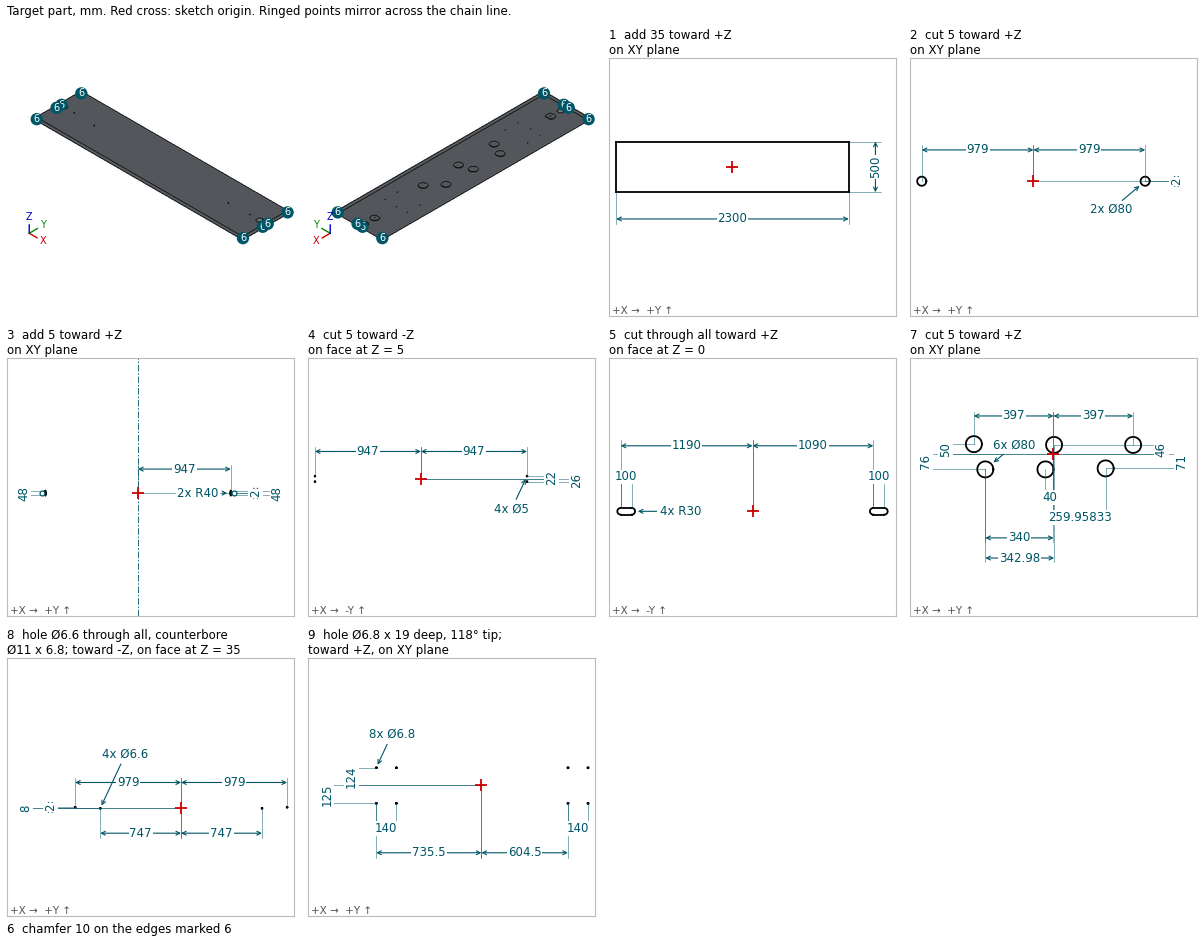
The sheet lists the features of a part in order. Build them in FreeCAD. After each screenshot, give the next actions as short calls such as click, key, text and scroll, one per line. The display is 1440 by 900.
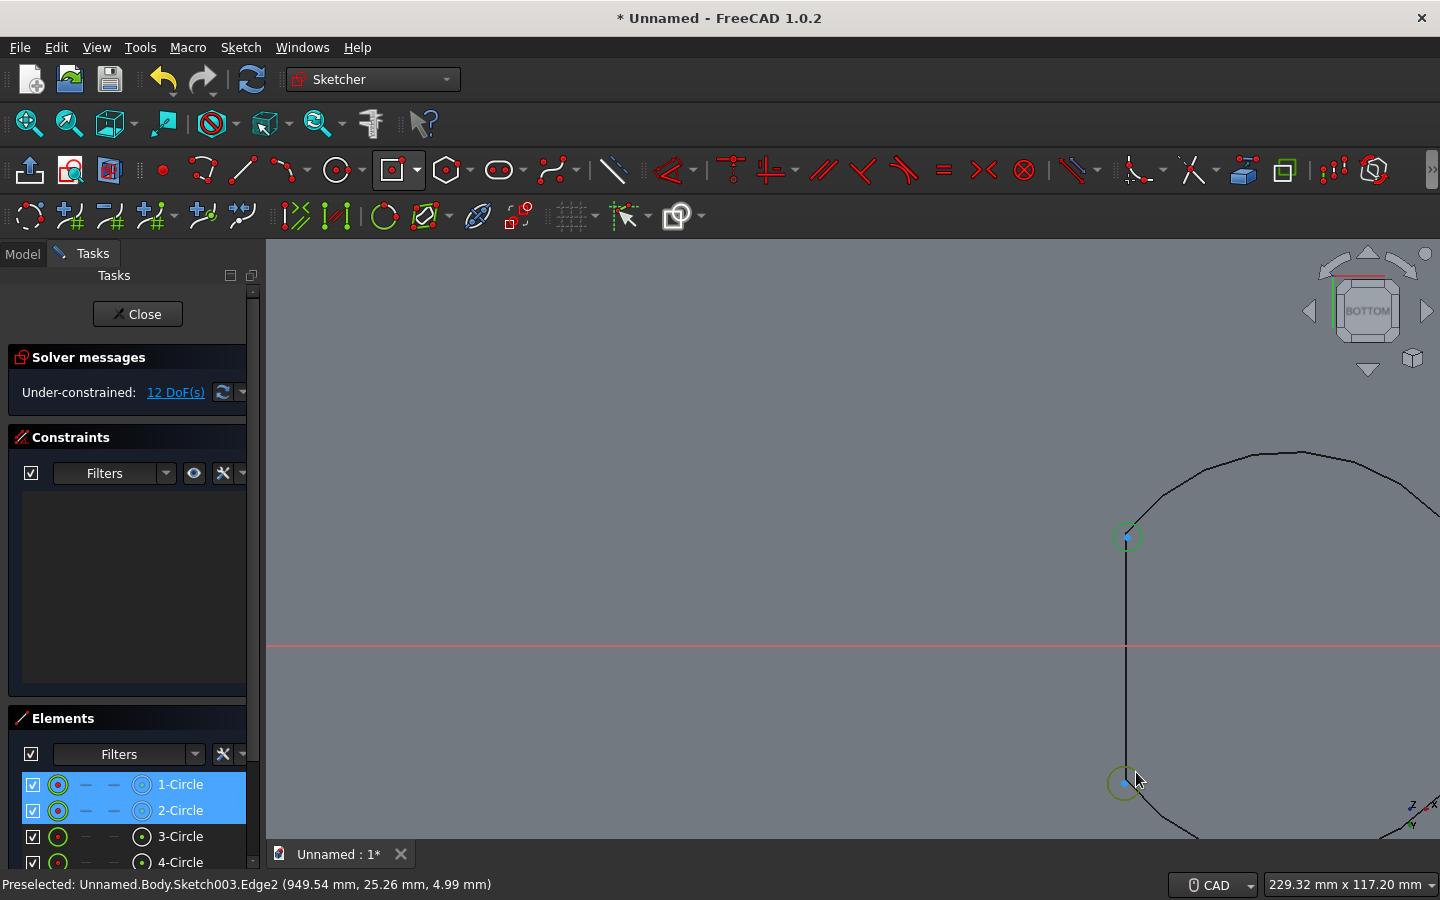
scroll(1146, 530, down, 13)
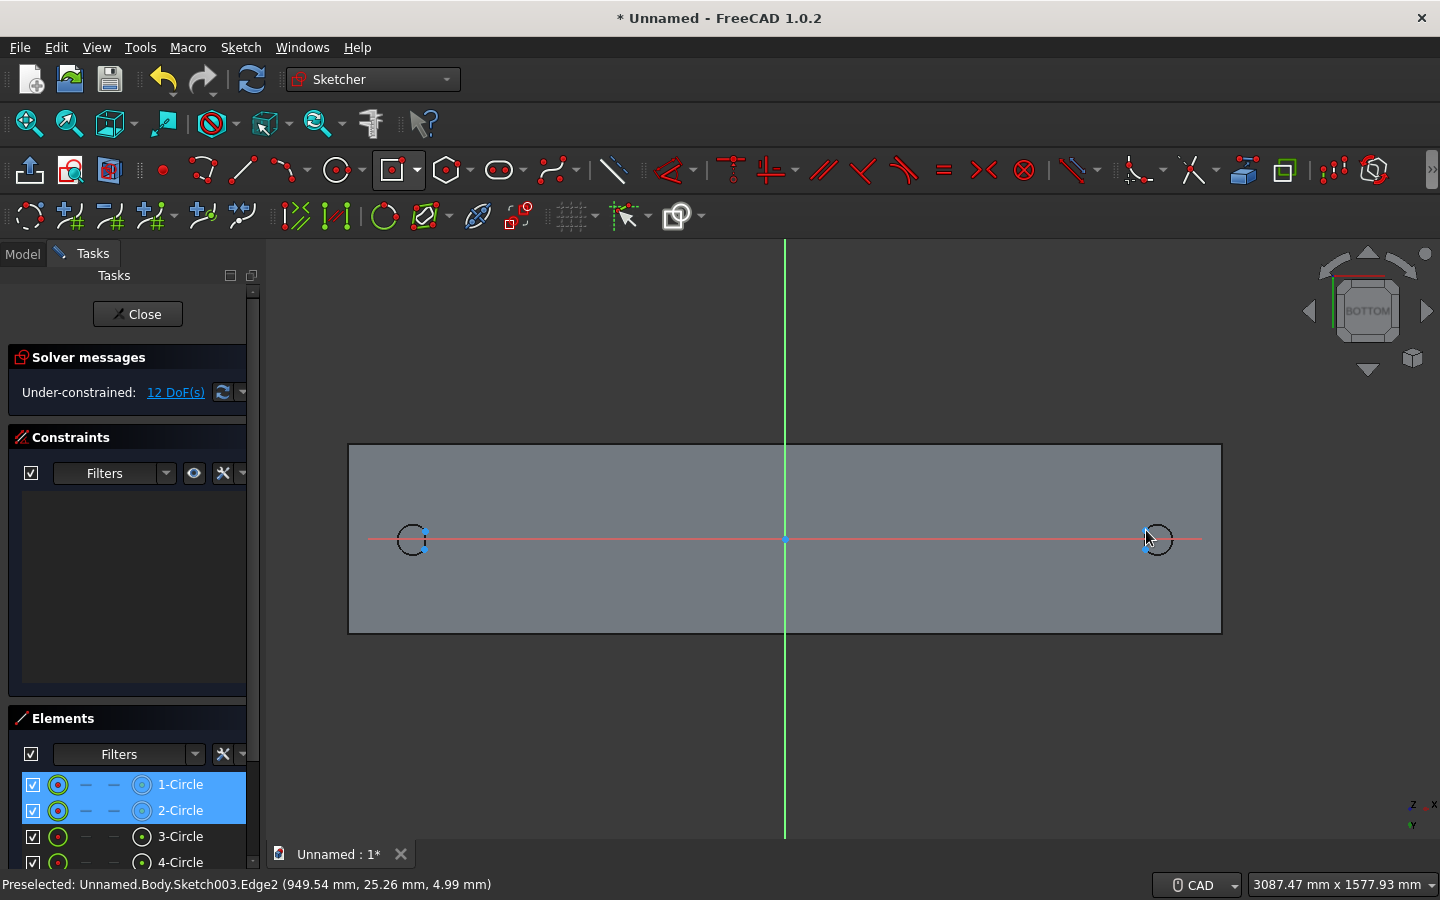
scroll(426, 530, up, 13)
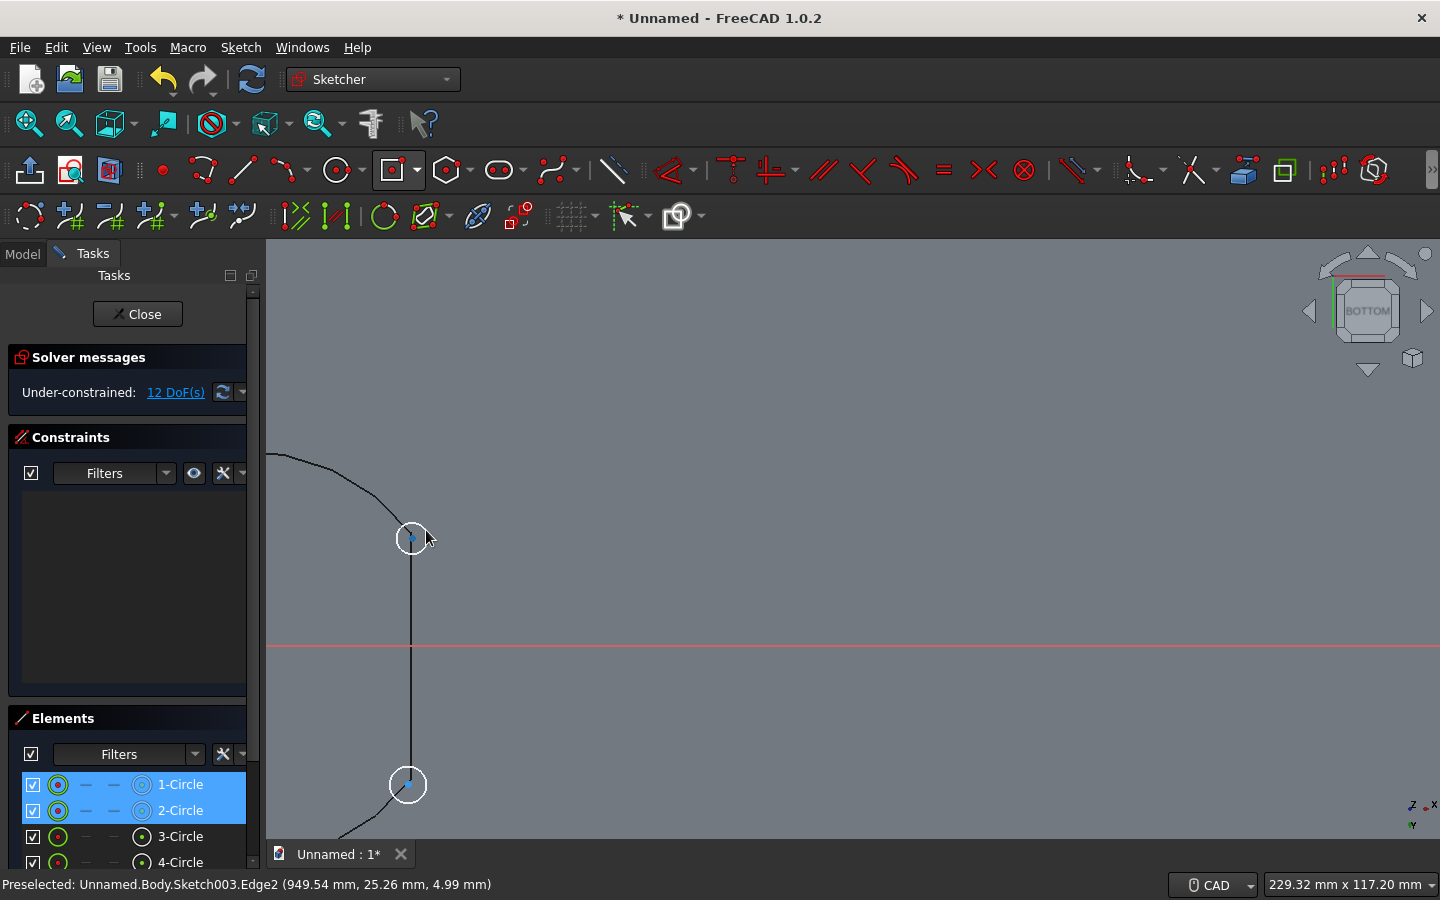
click(423, 527)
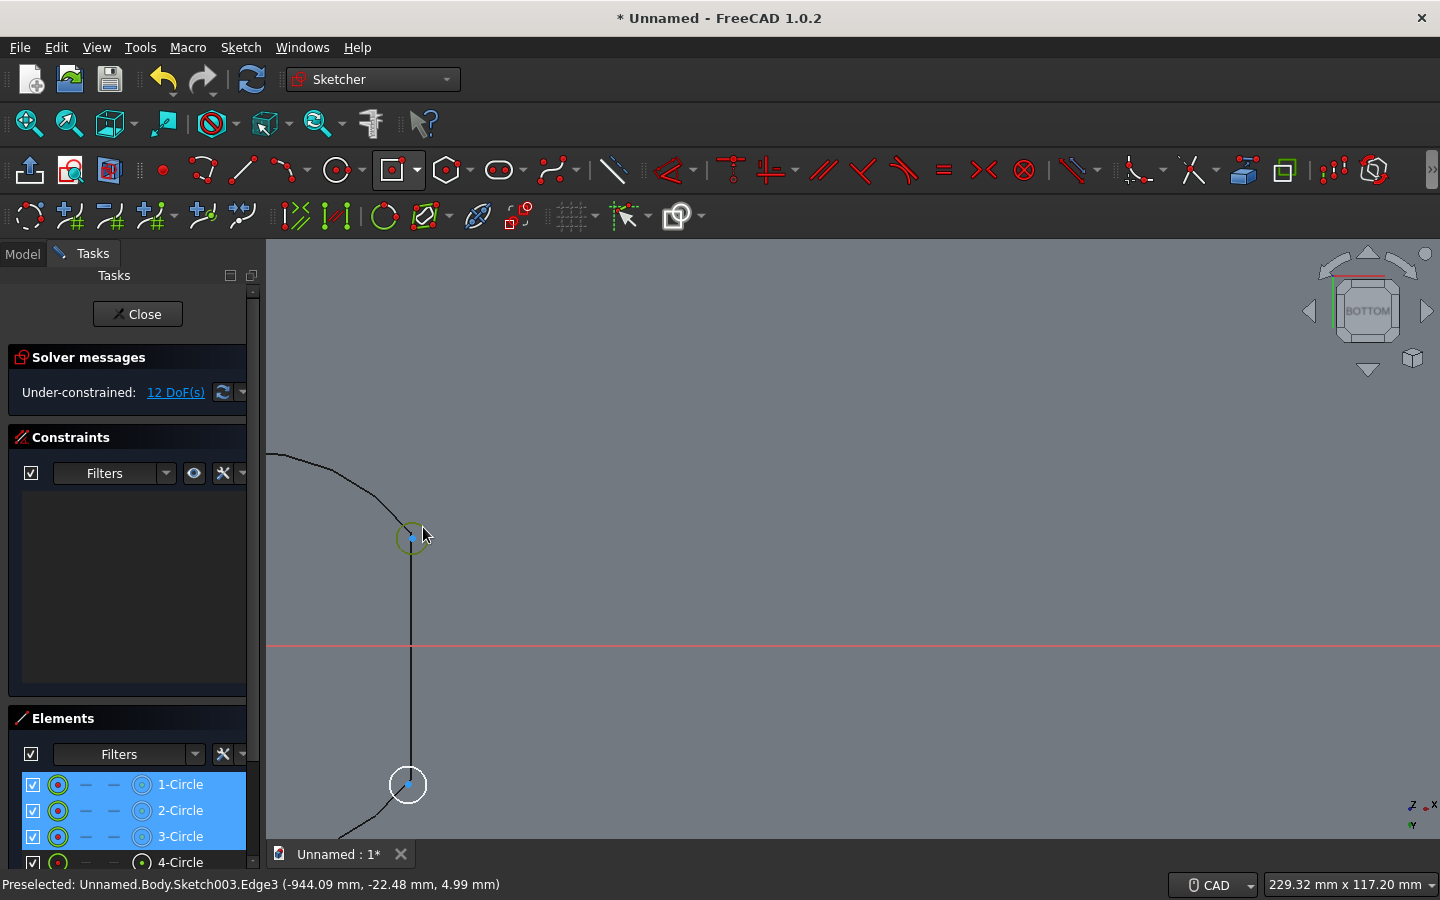
click(421, 772)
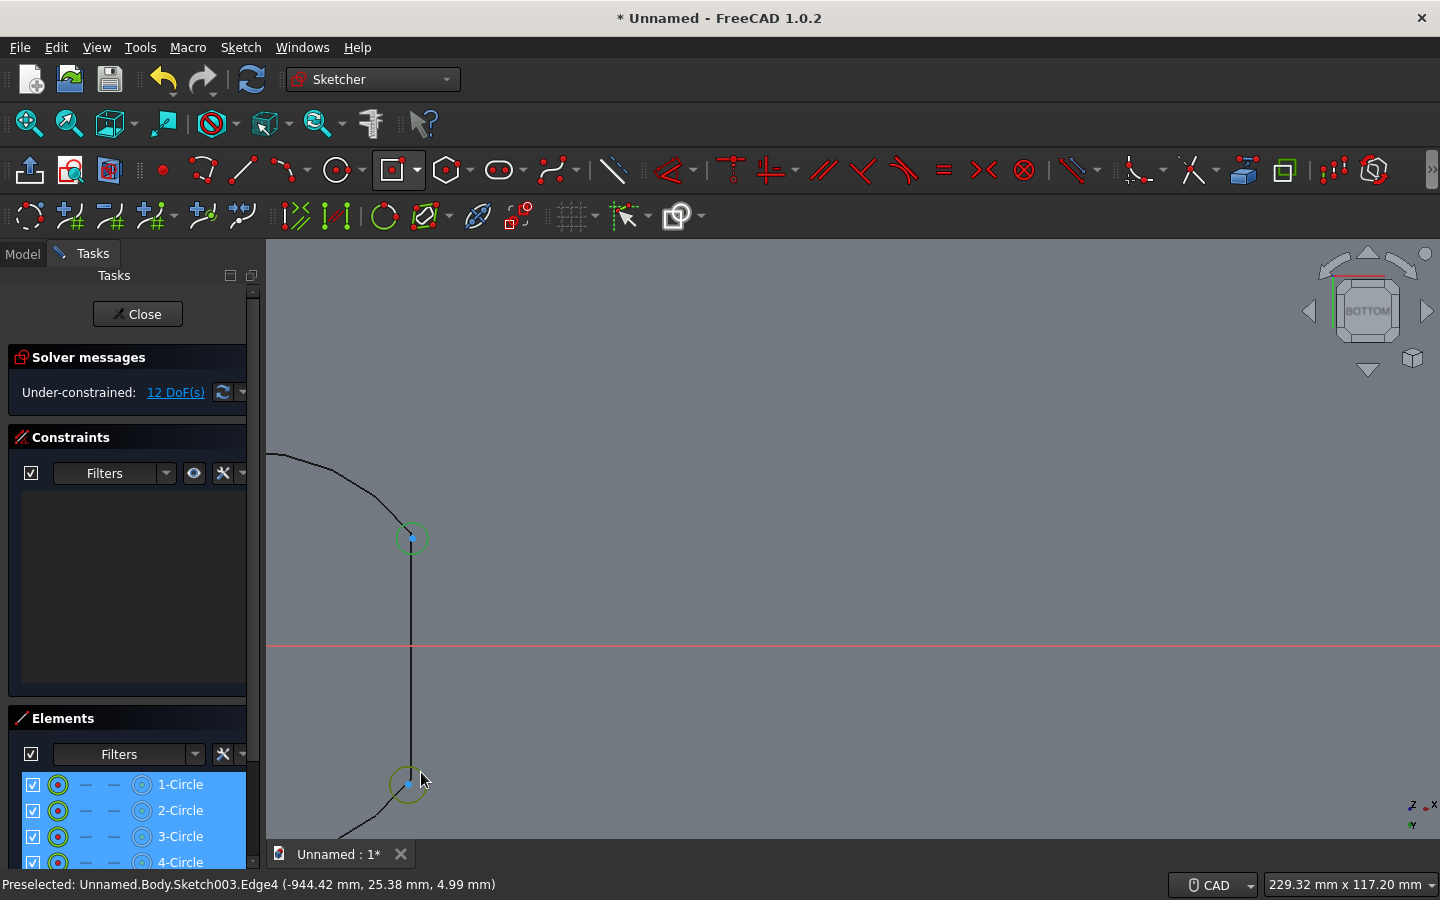
click(944, 170)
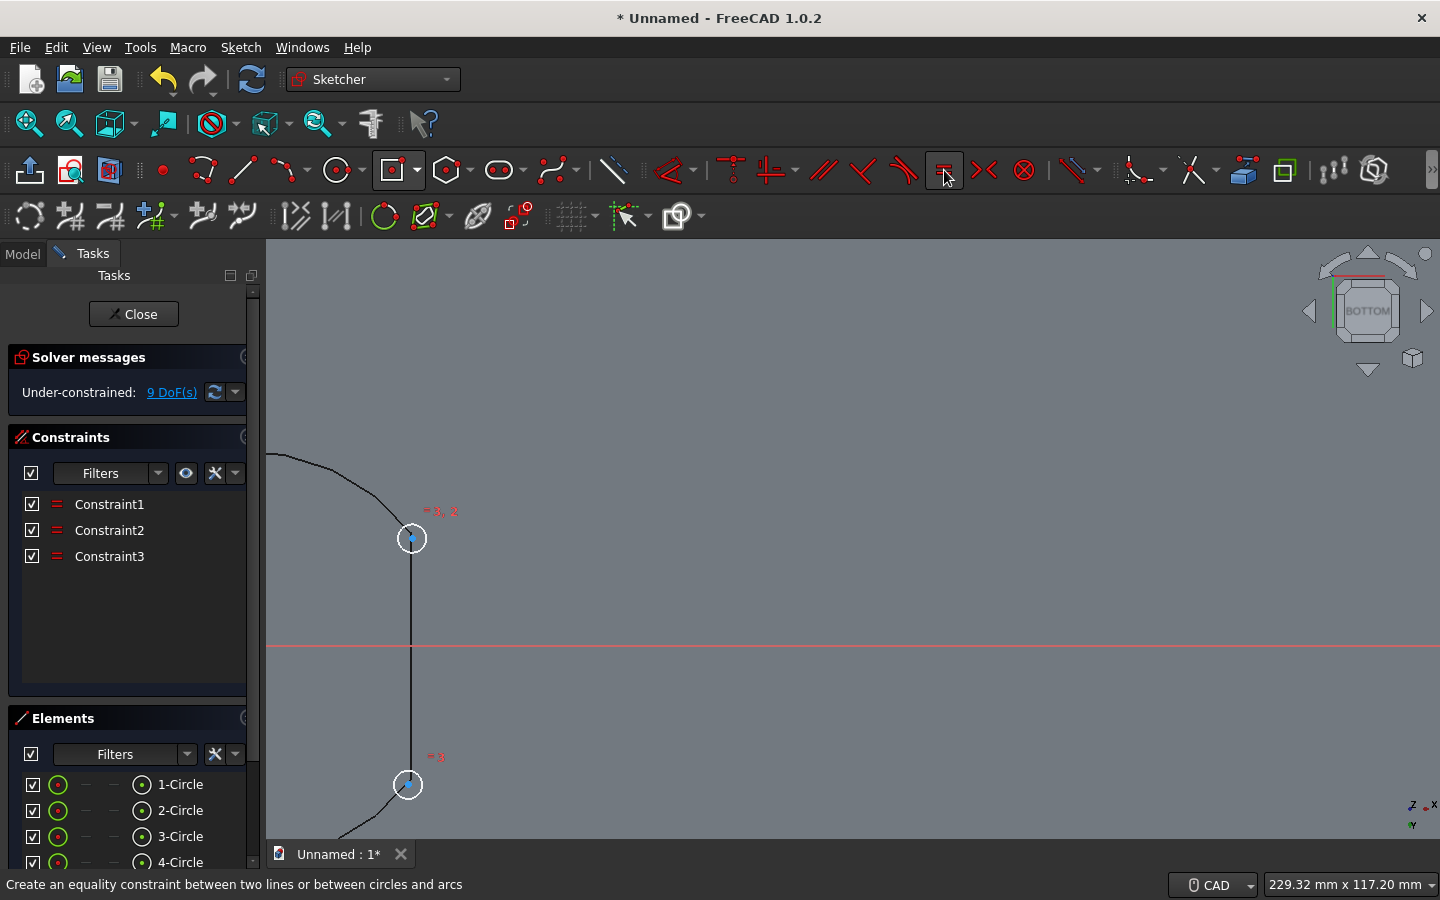
scroll(425, 530, down, 13)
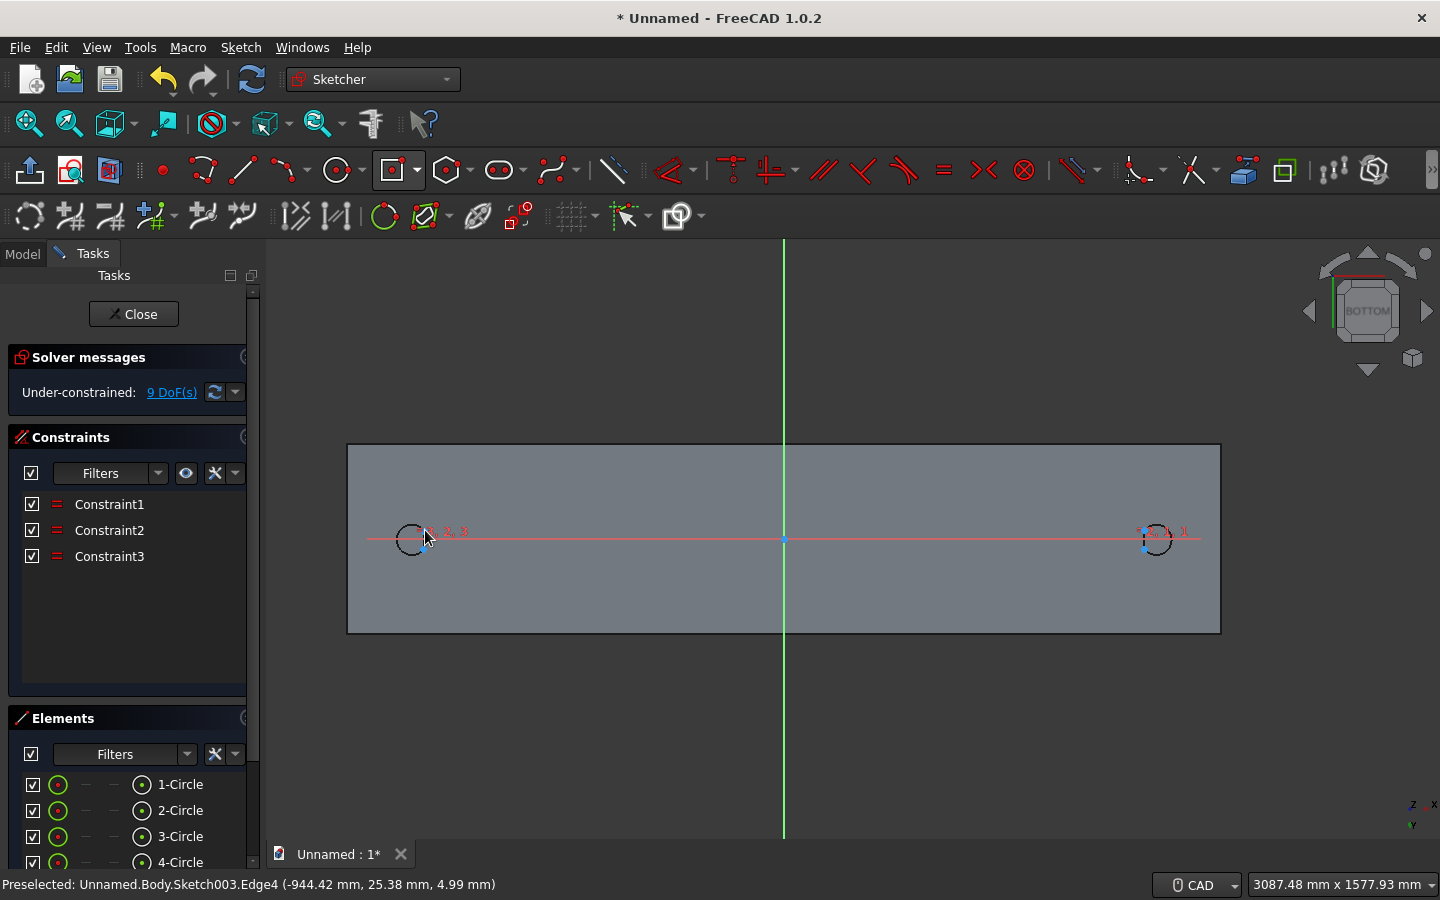
click(1144, 531)